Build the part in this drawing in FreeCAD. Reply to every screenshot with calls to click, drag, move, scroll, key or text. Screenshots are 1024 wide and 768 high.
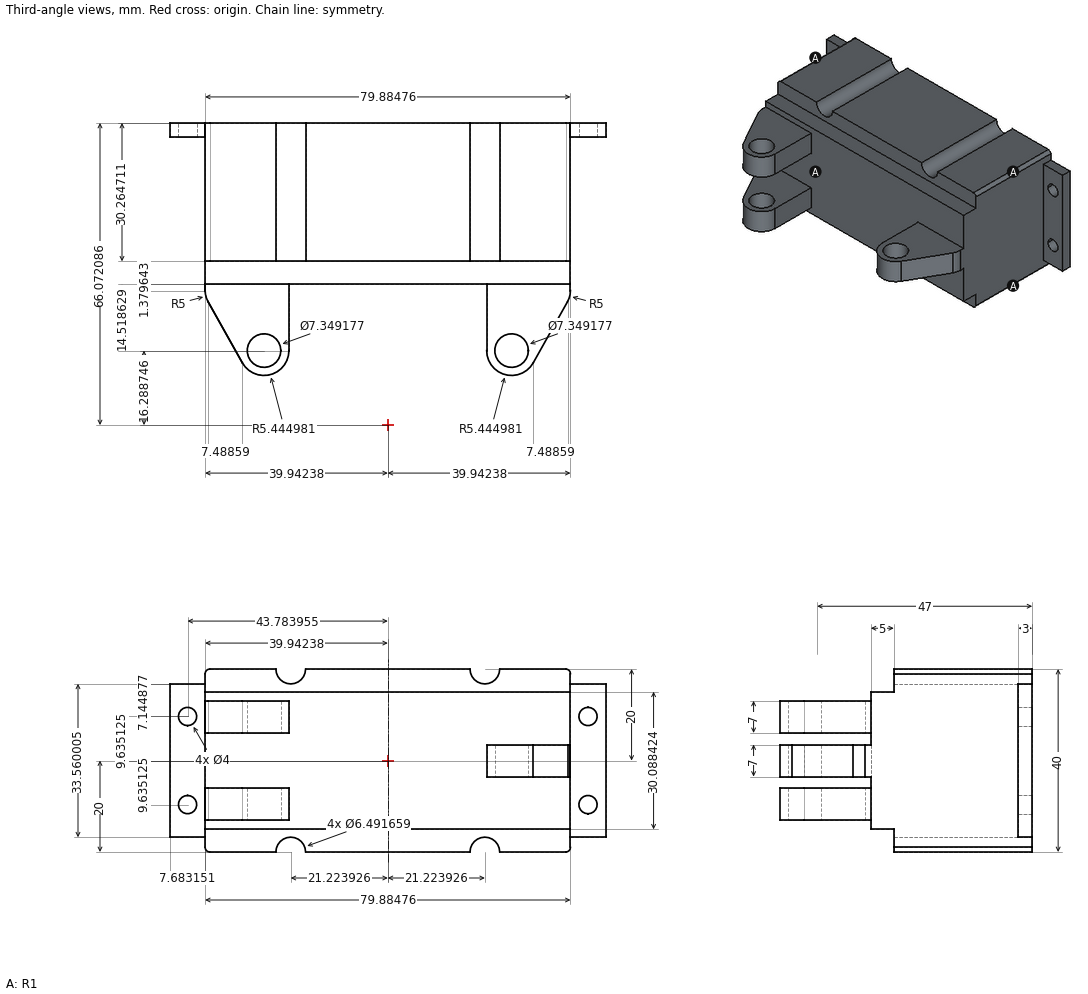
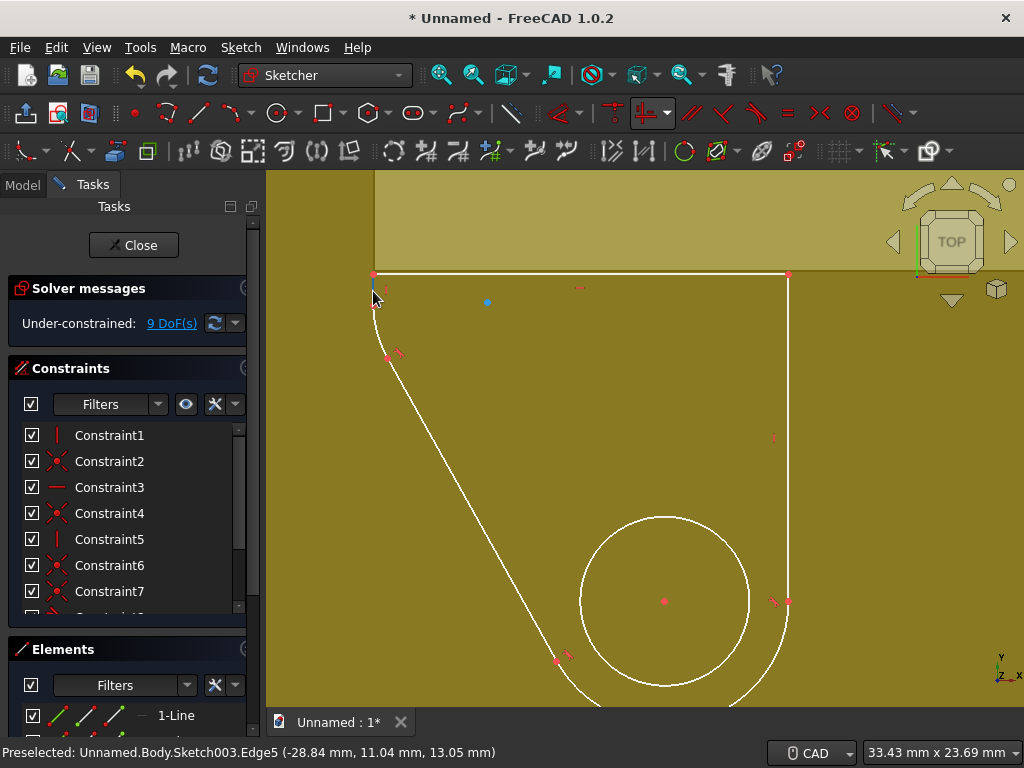
click(373, 290)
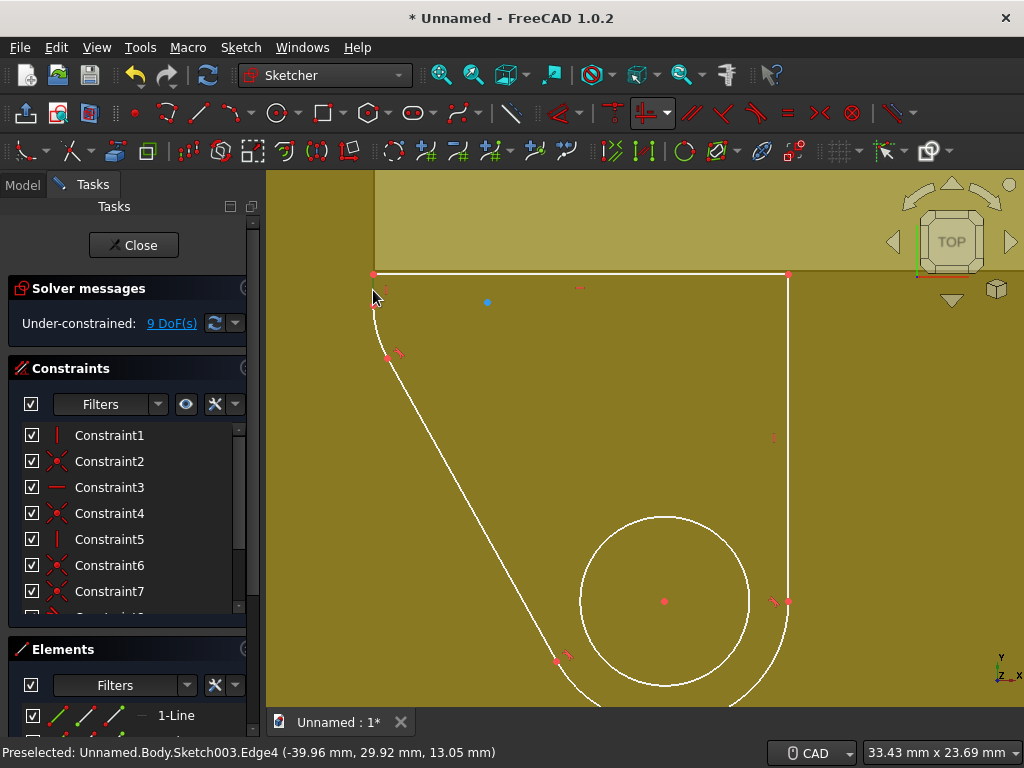
click(375, 322)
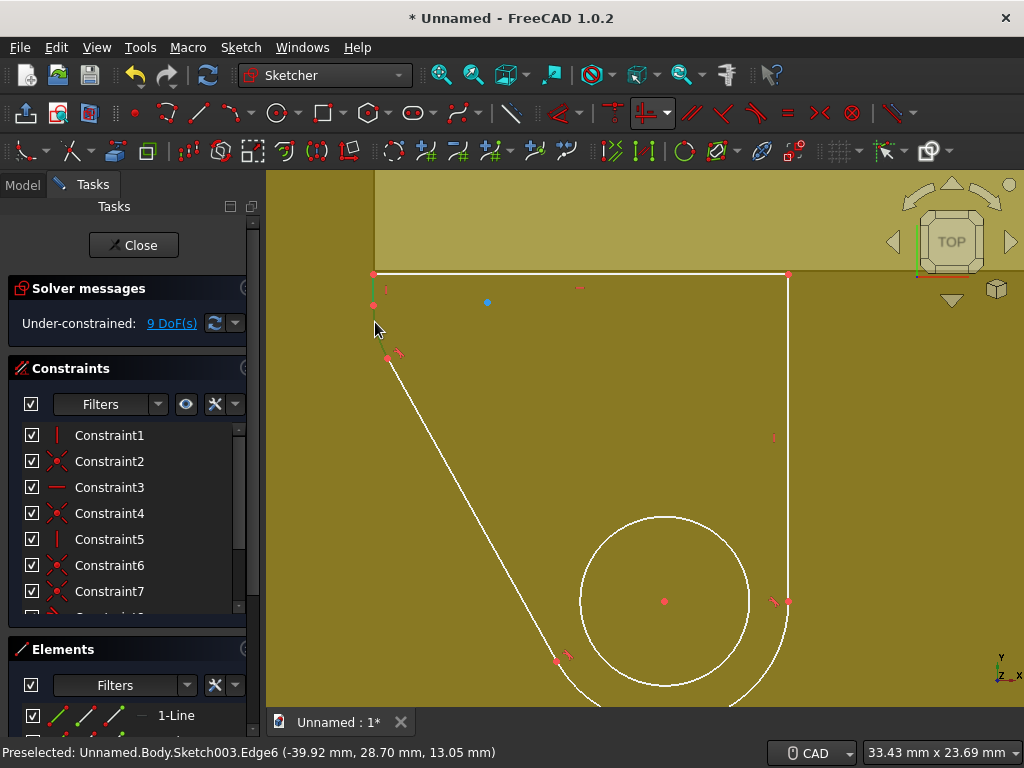
click(756, 114)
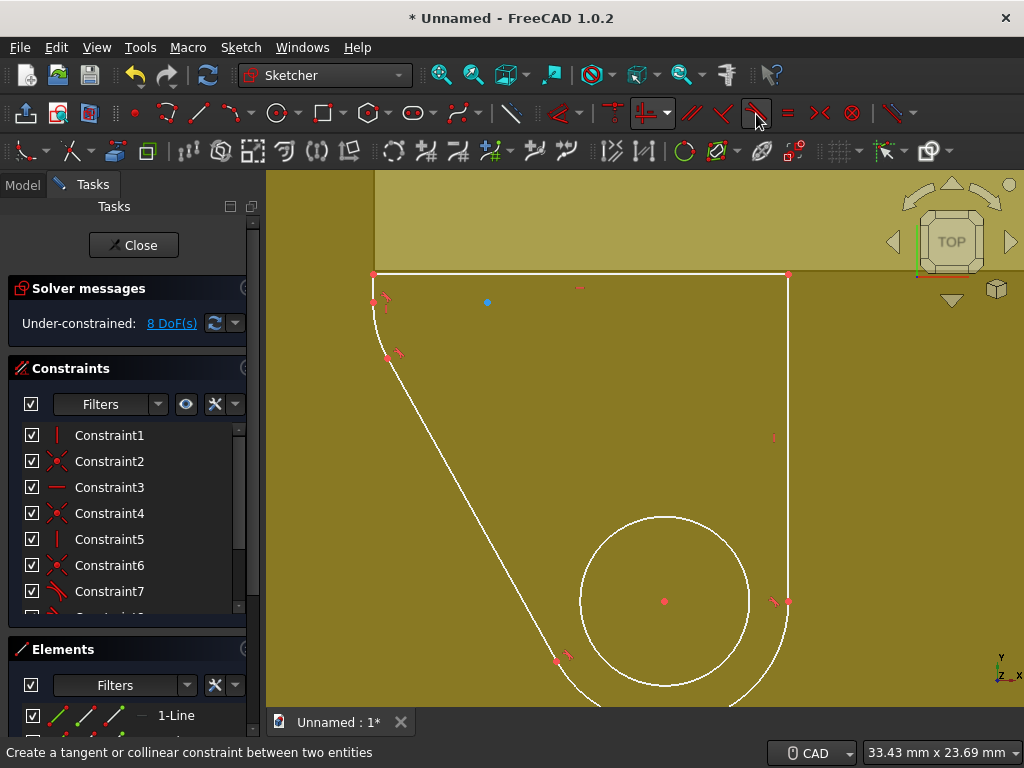
click(558, 114)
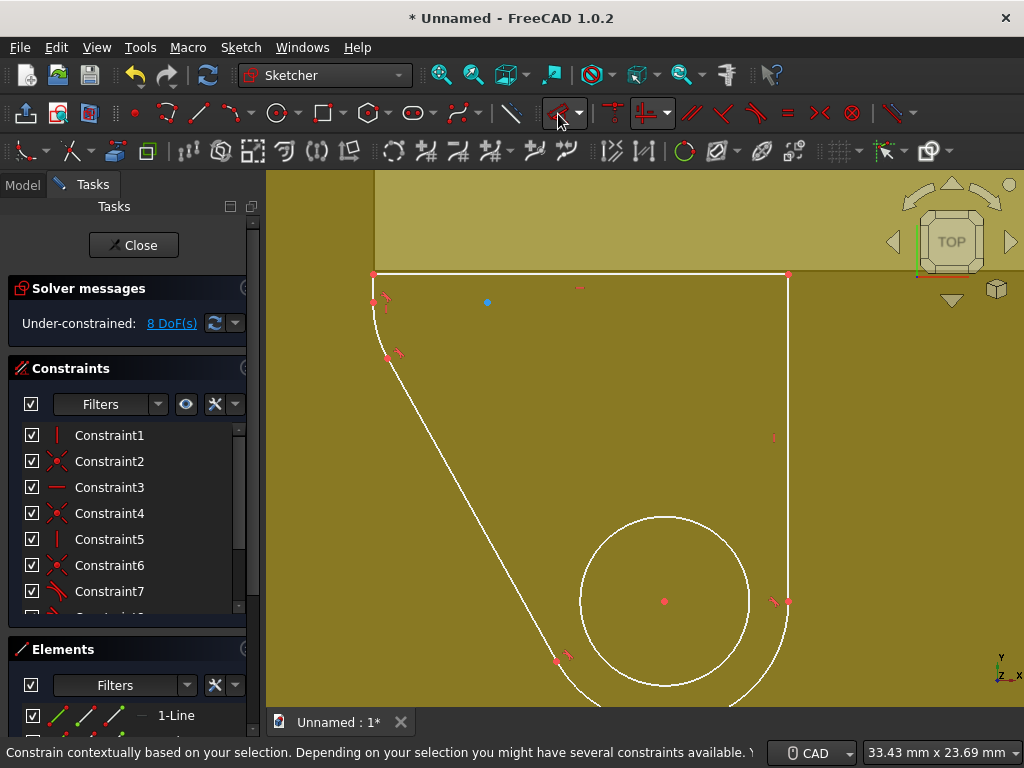
click(772, 663)
click(800, 679)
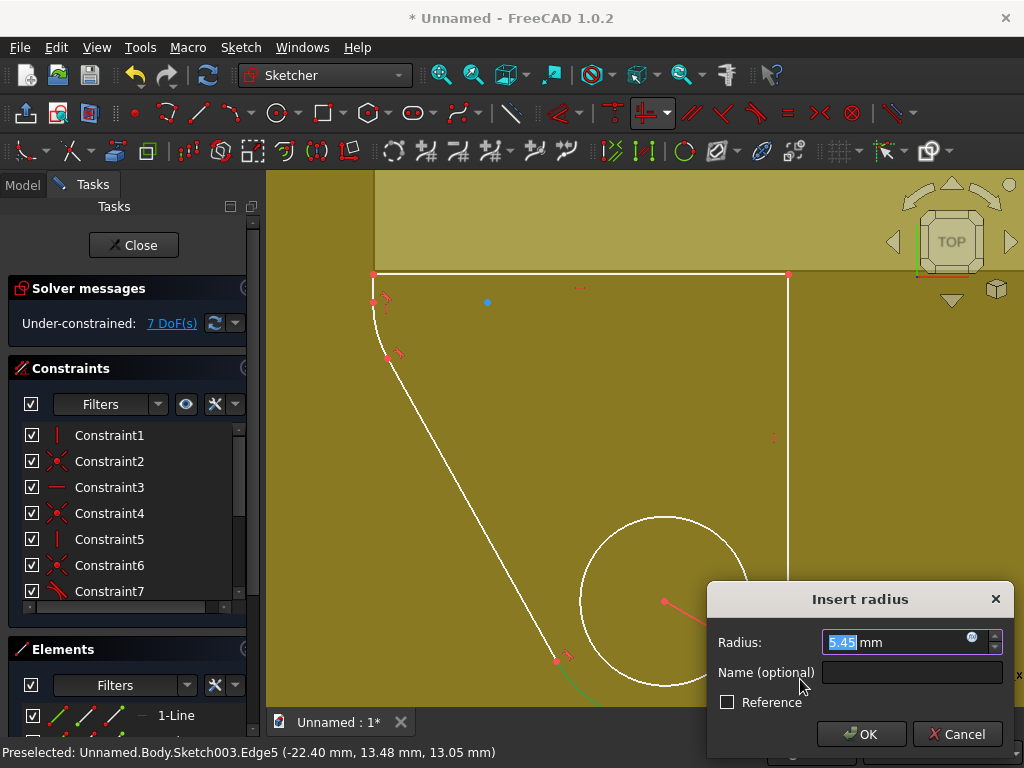
text(5.444981)
key(Return)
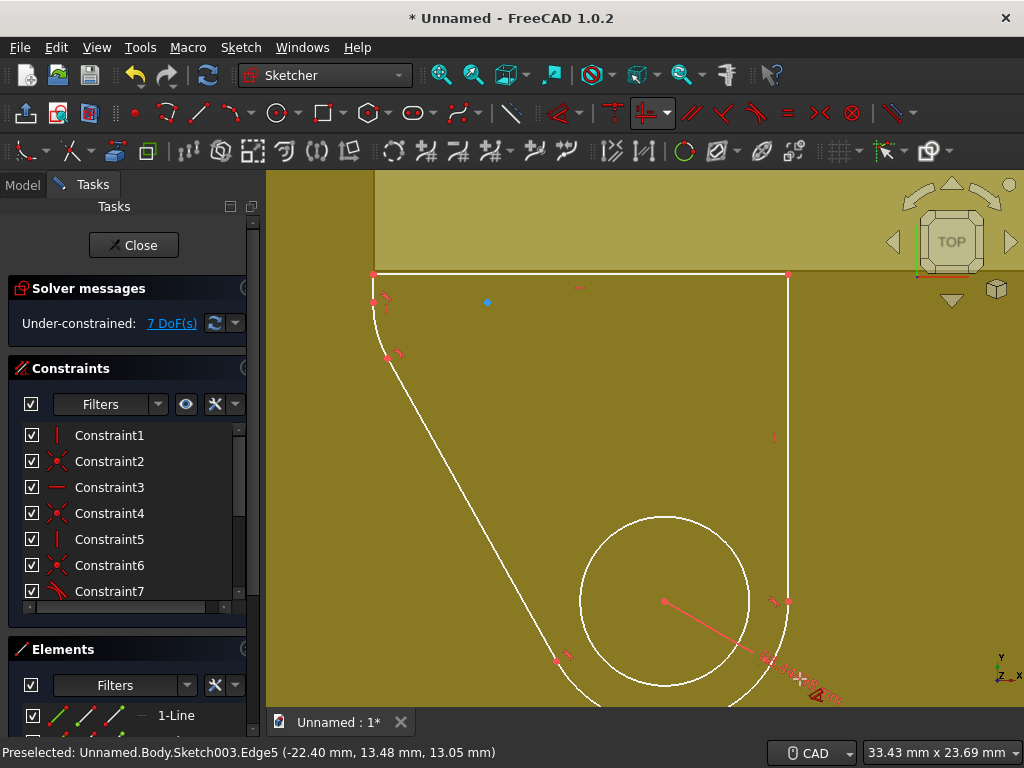
click(375, 320)
click(343, 325)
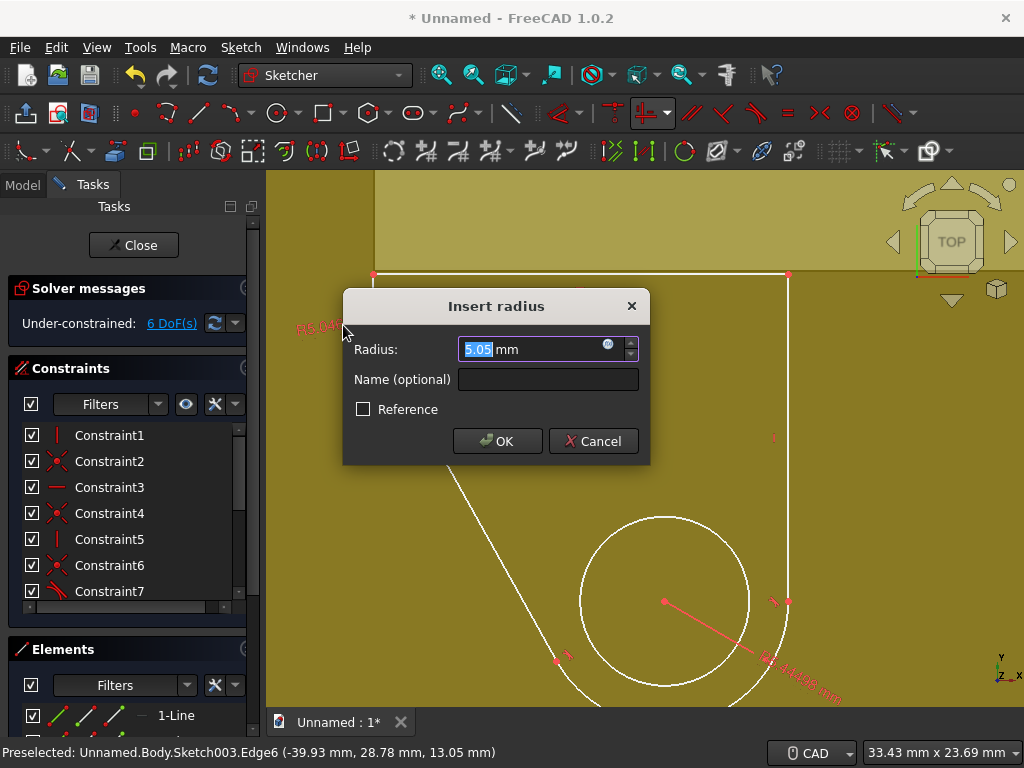
text(5)
key(Return)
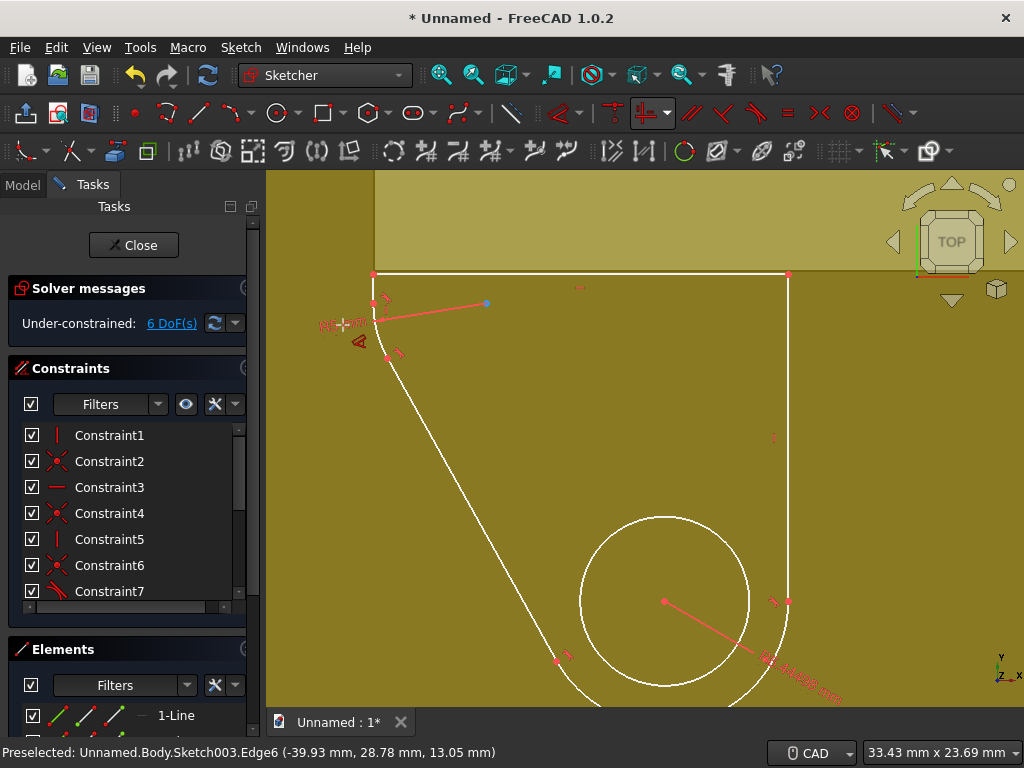
click(724, 541)
click(746, 518)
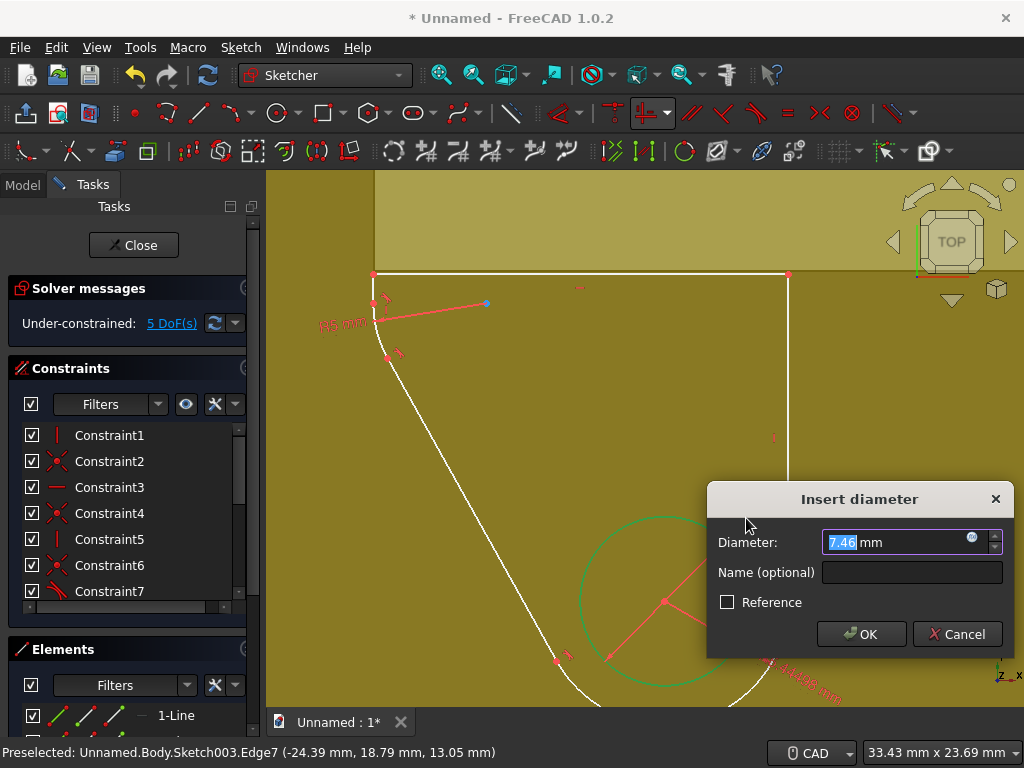
text(7.349177)
key(Return)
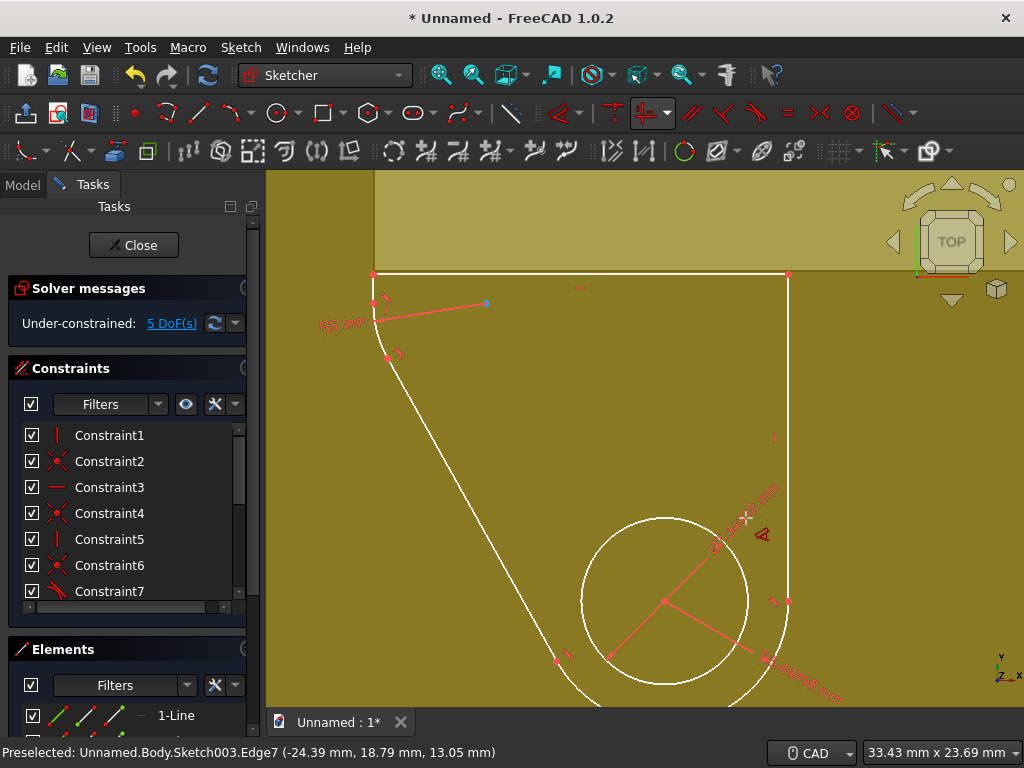
scroll(373, 286, up, 2)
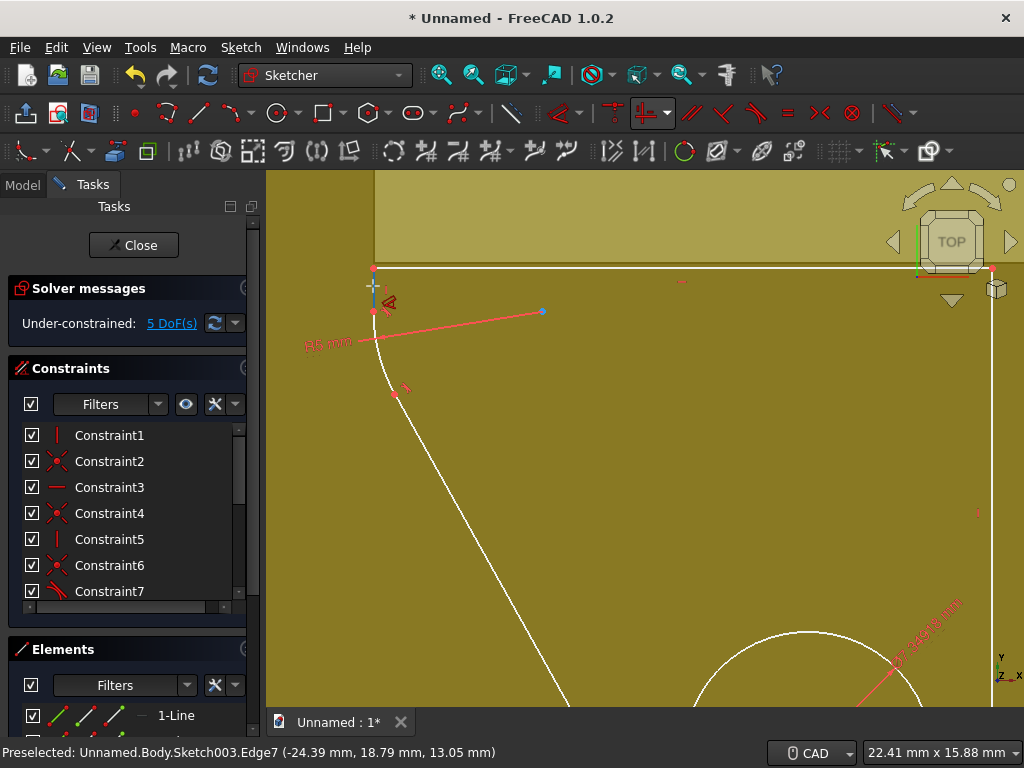
click(374, 286)
click(340, 290)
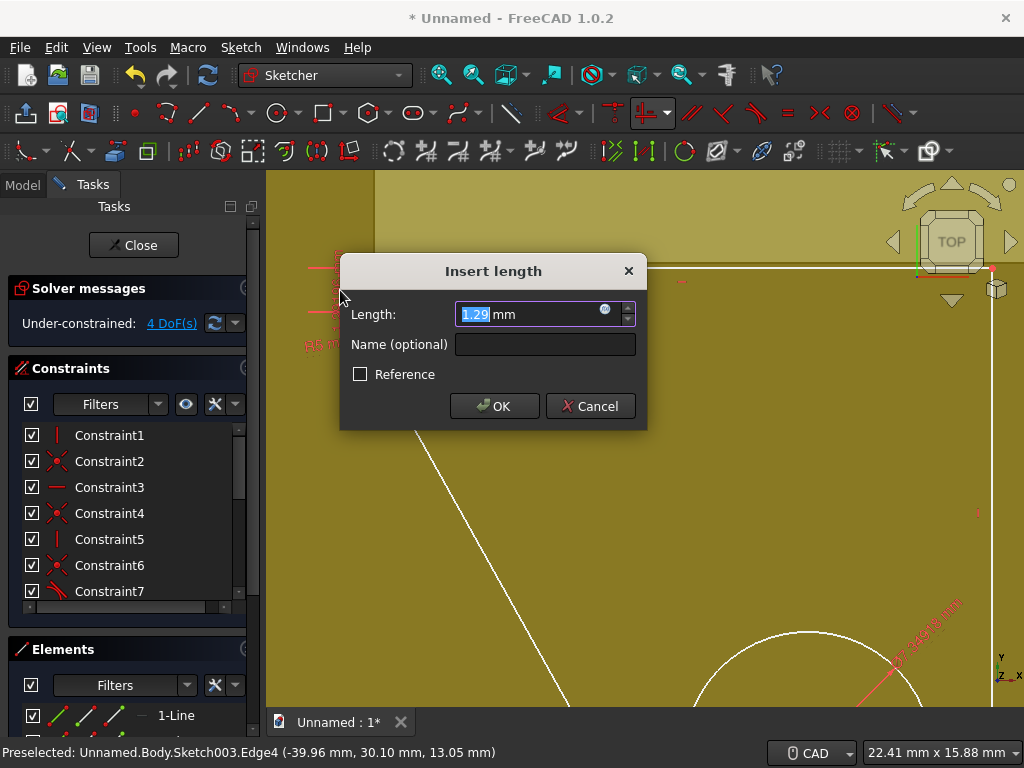
text(1.379643)
key(Return)